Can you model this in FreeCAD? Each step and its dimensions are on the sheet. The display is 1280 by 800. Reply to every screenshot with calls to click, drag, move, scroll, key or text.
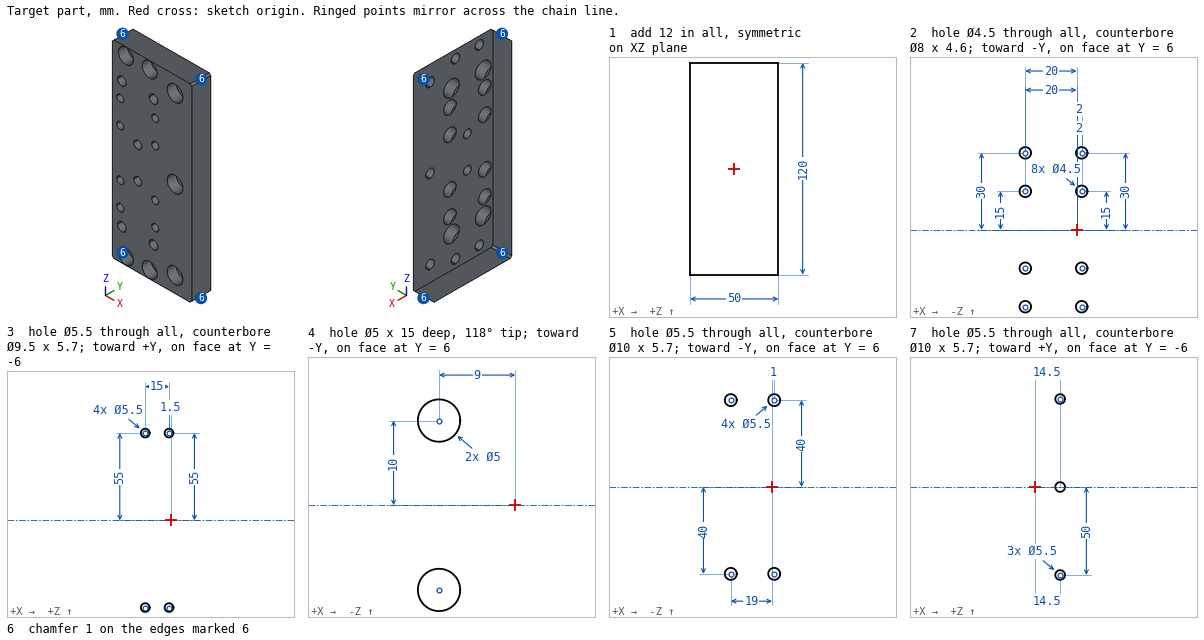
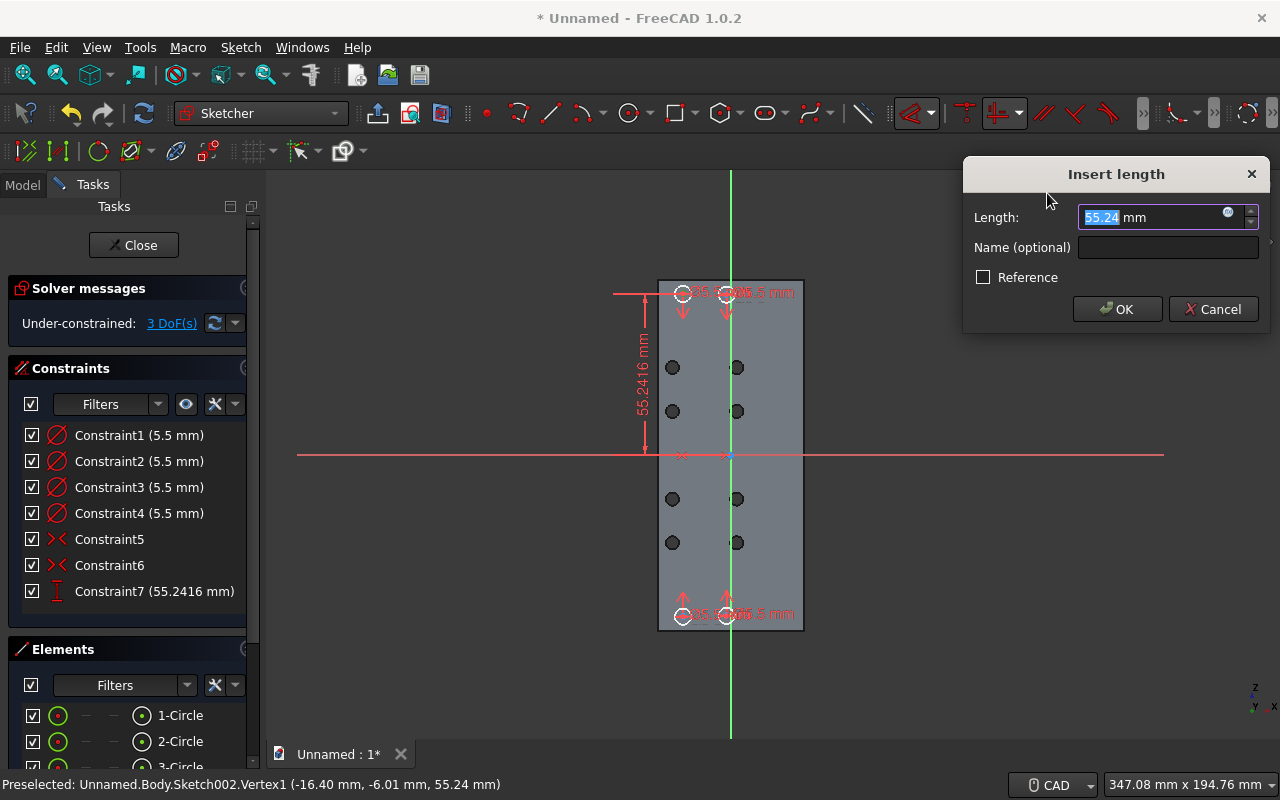
text(55)
key(Return)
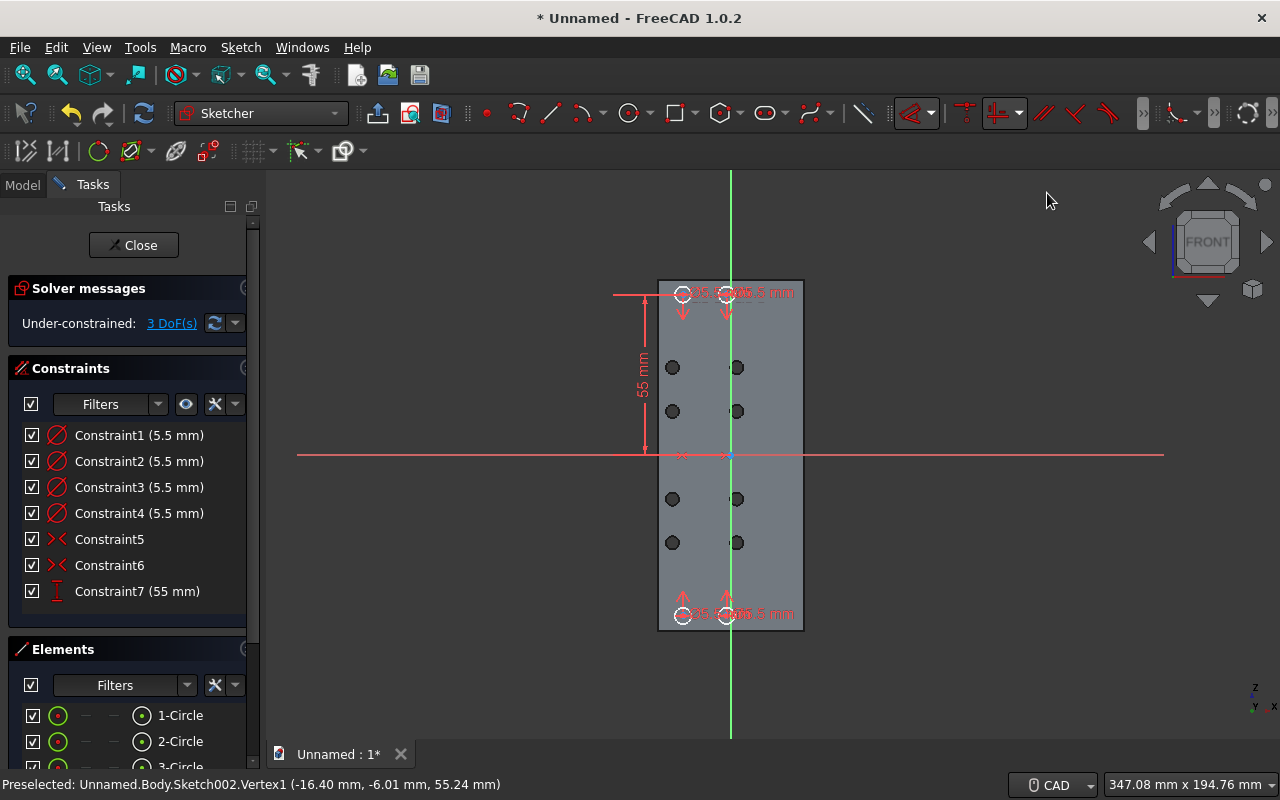
click(727, 295)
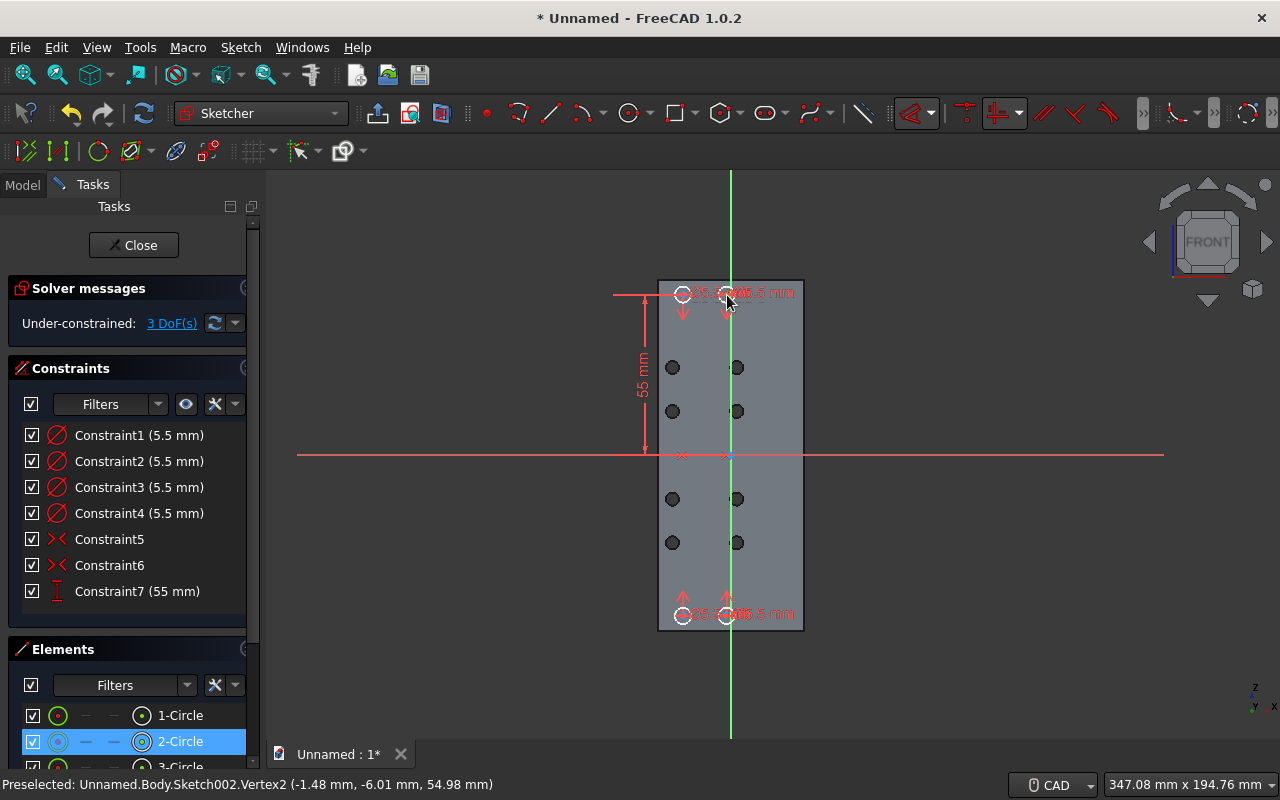
click(934, 114)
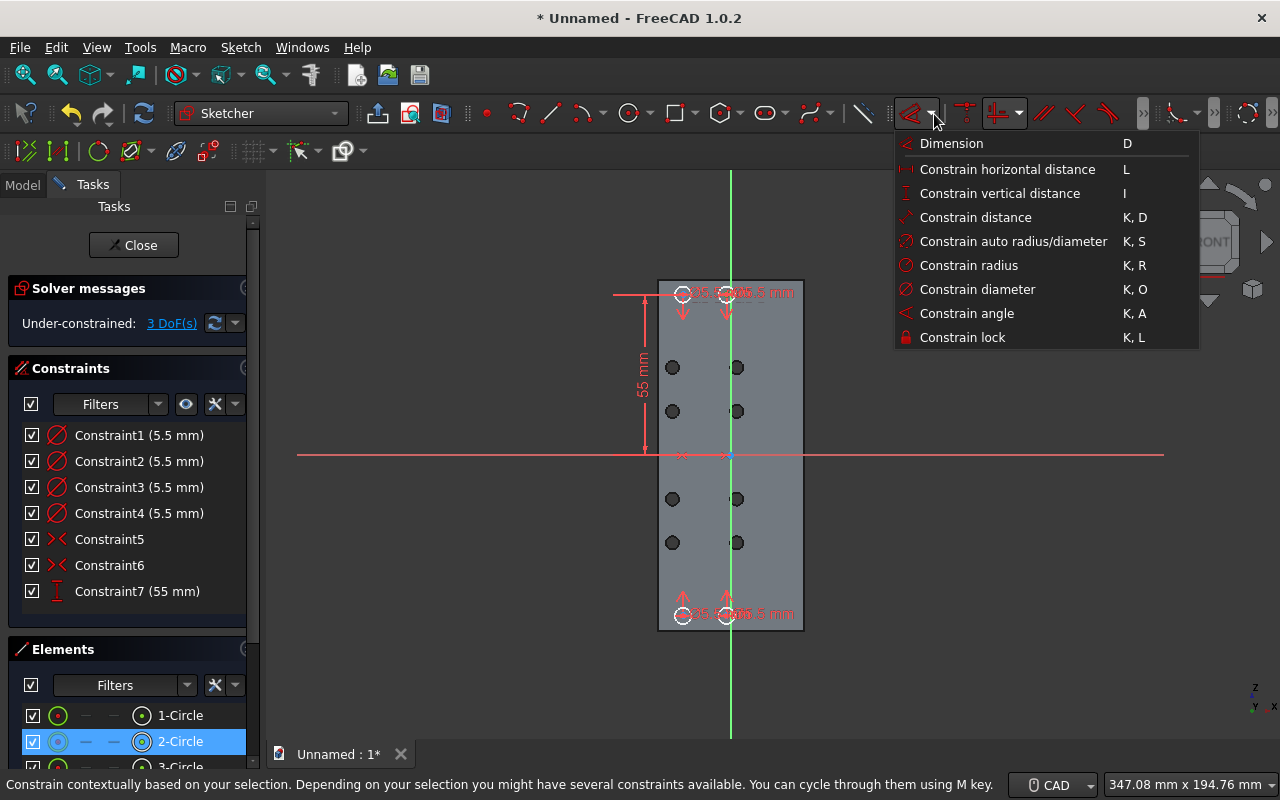
click(1047, 193)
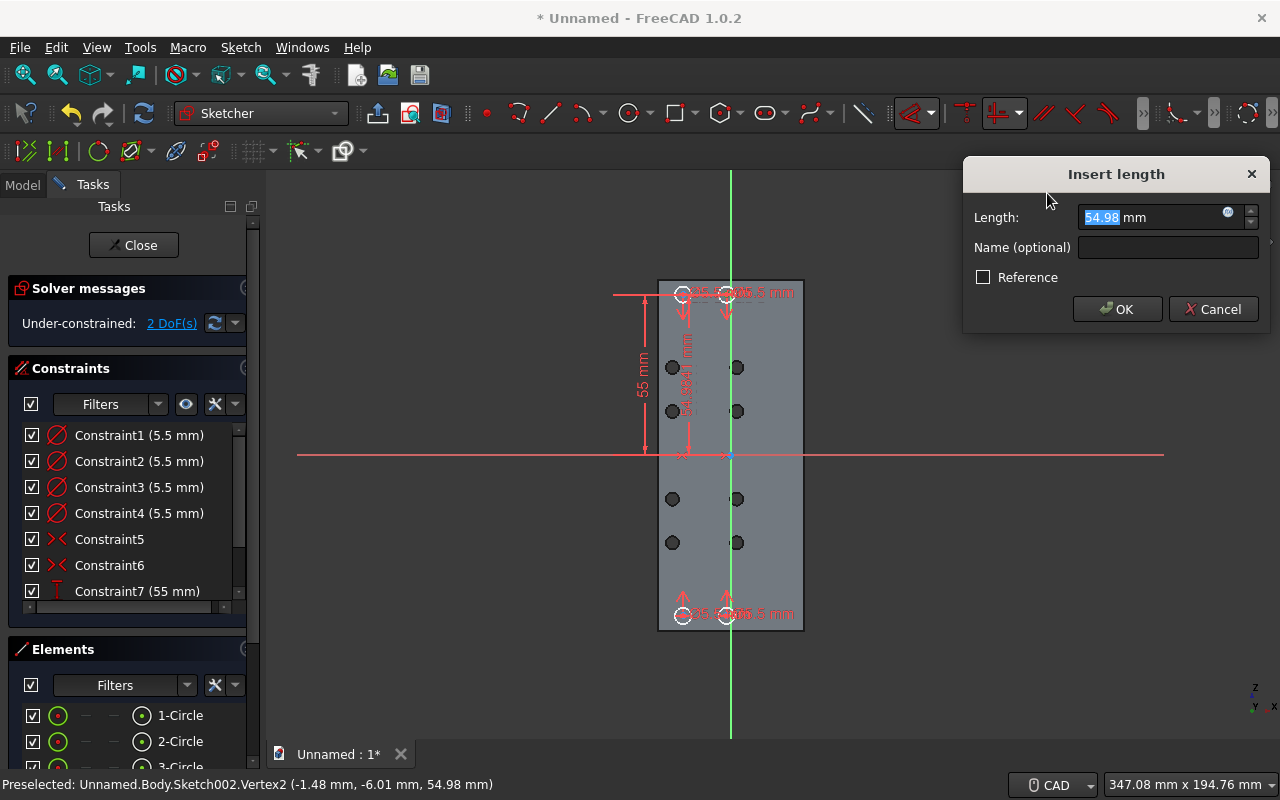
text(55)
key(Return)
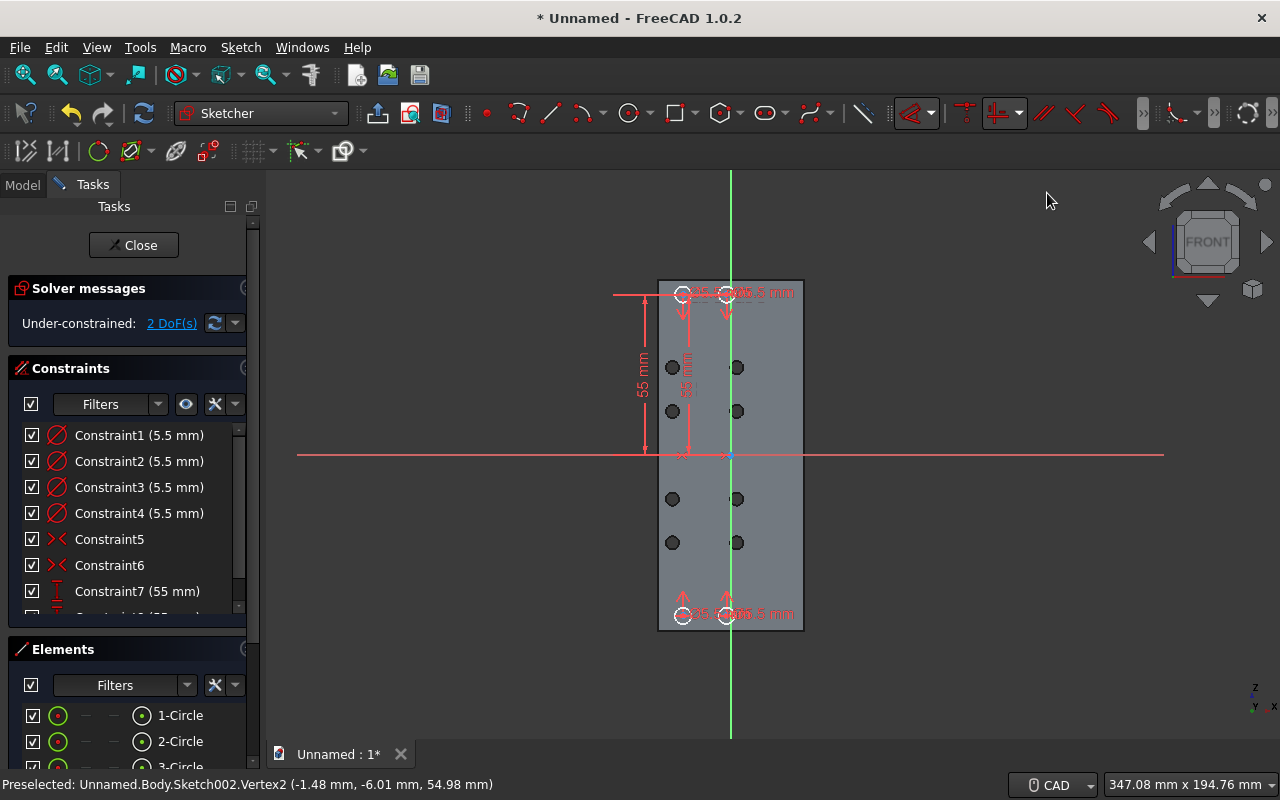
scroll(727, 295, up, 12)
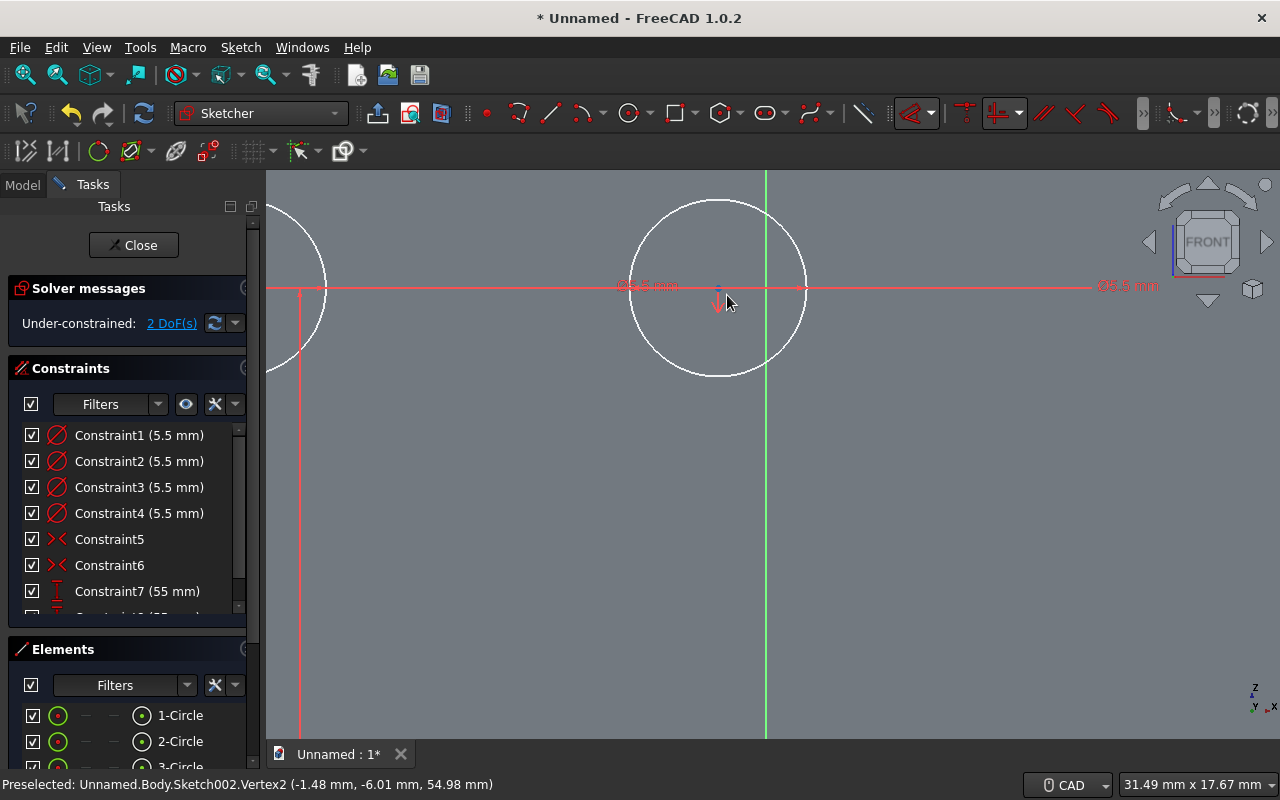
click(718, 288)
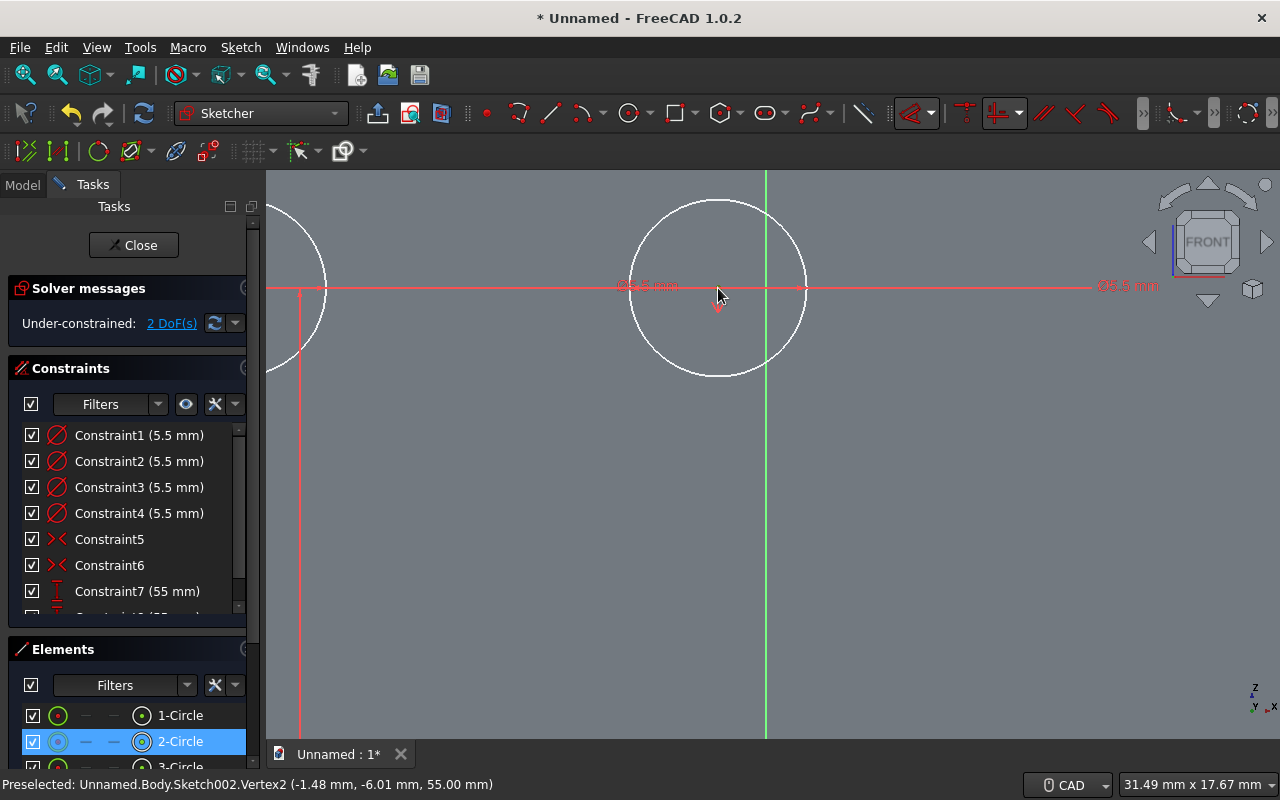
click(934, 114)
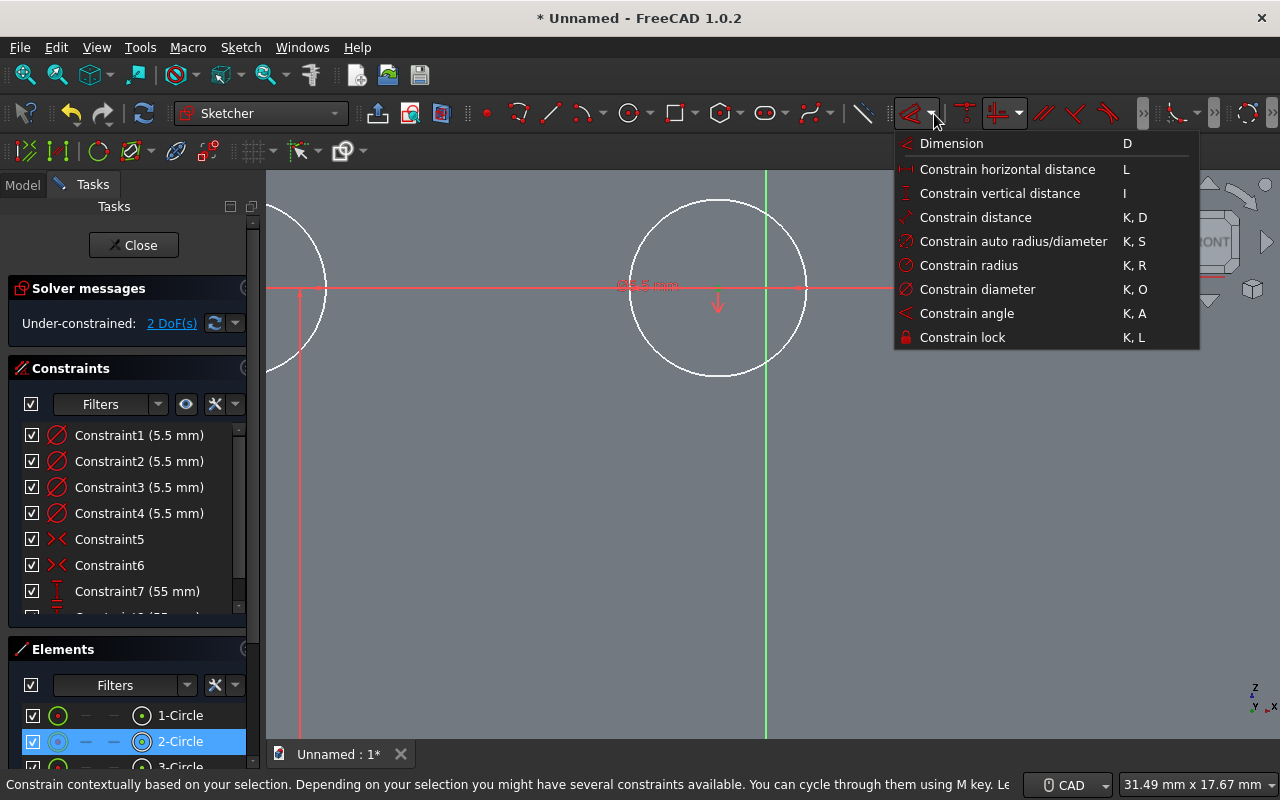
click(1047, 169)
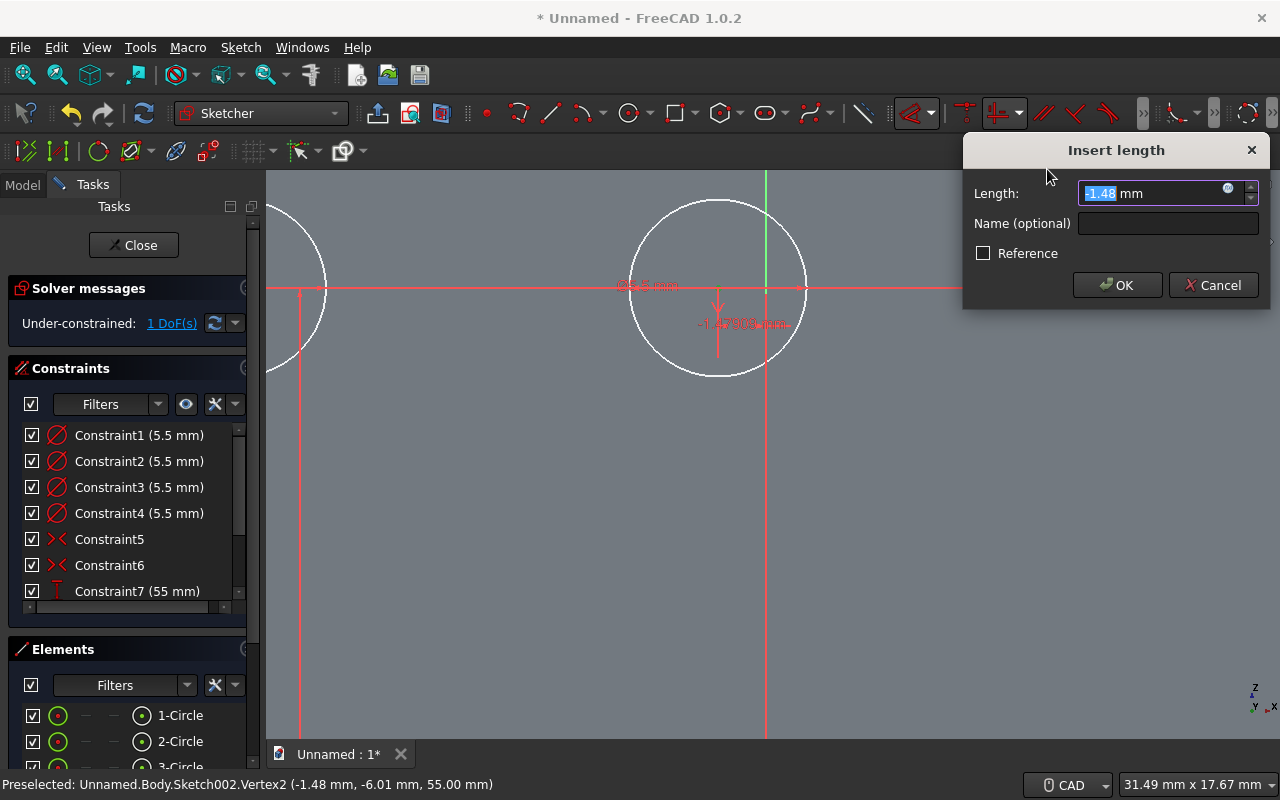
text(-1.5)
key(Return)